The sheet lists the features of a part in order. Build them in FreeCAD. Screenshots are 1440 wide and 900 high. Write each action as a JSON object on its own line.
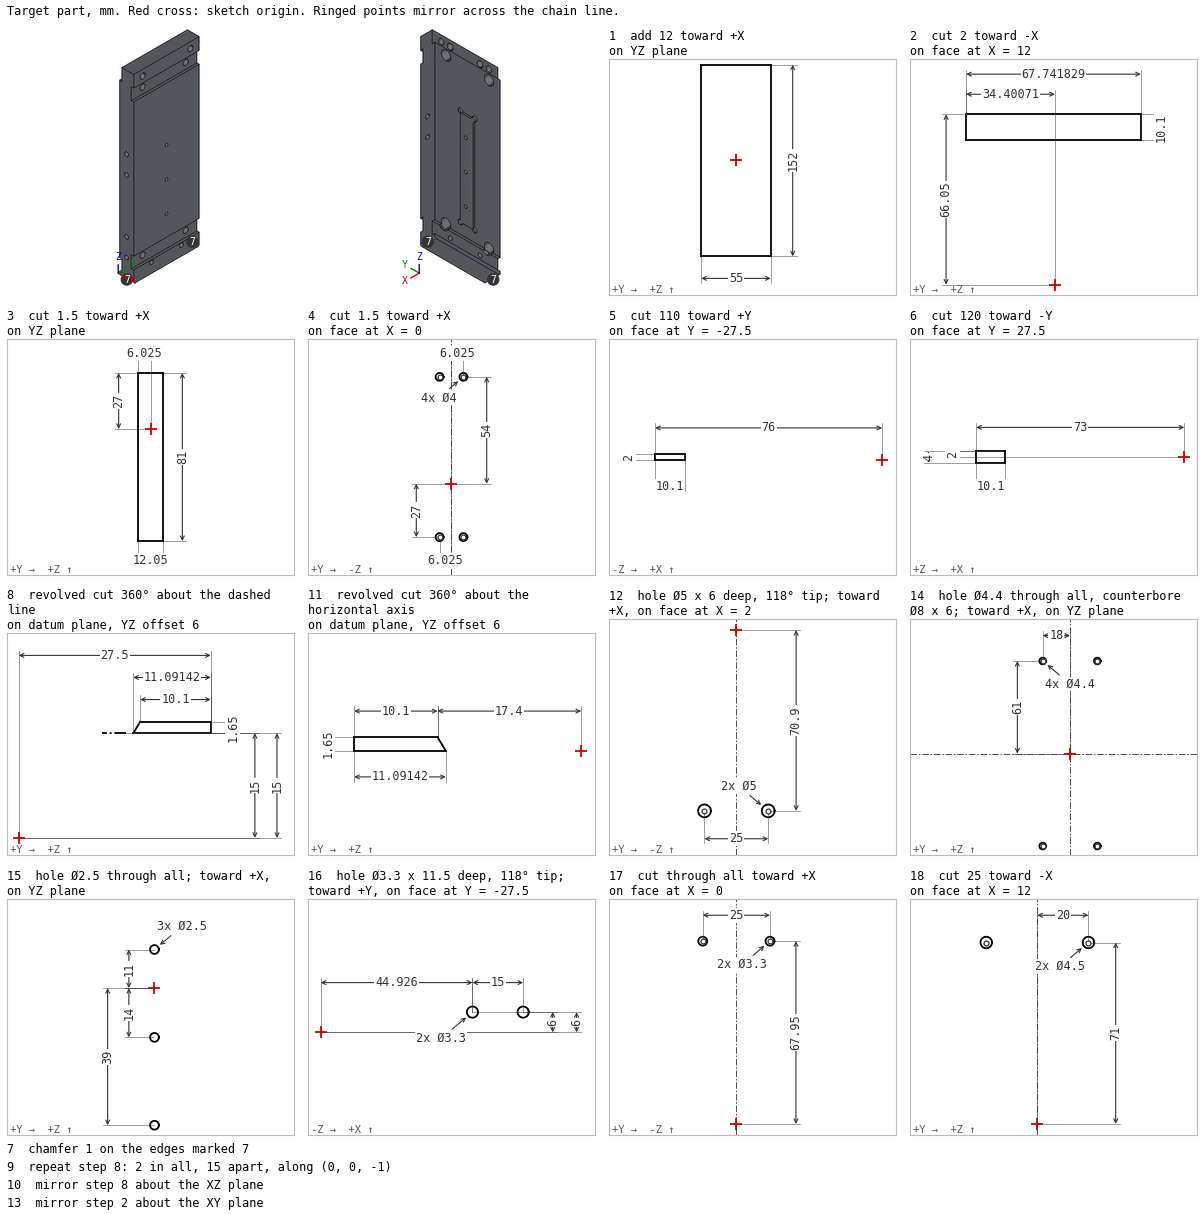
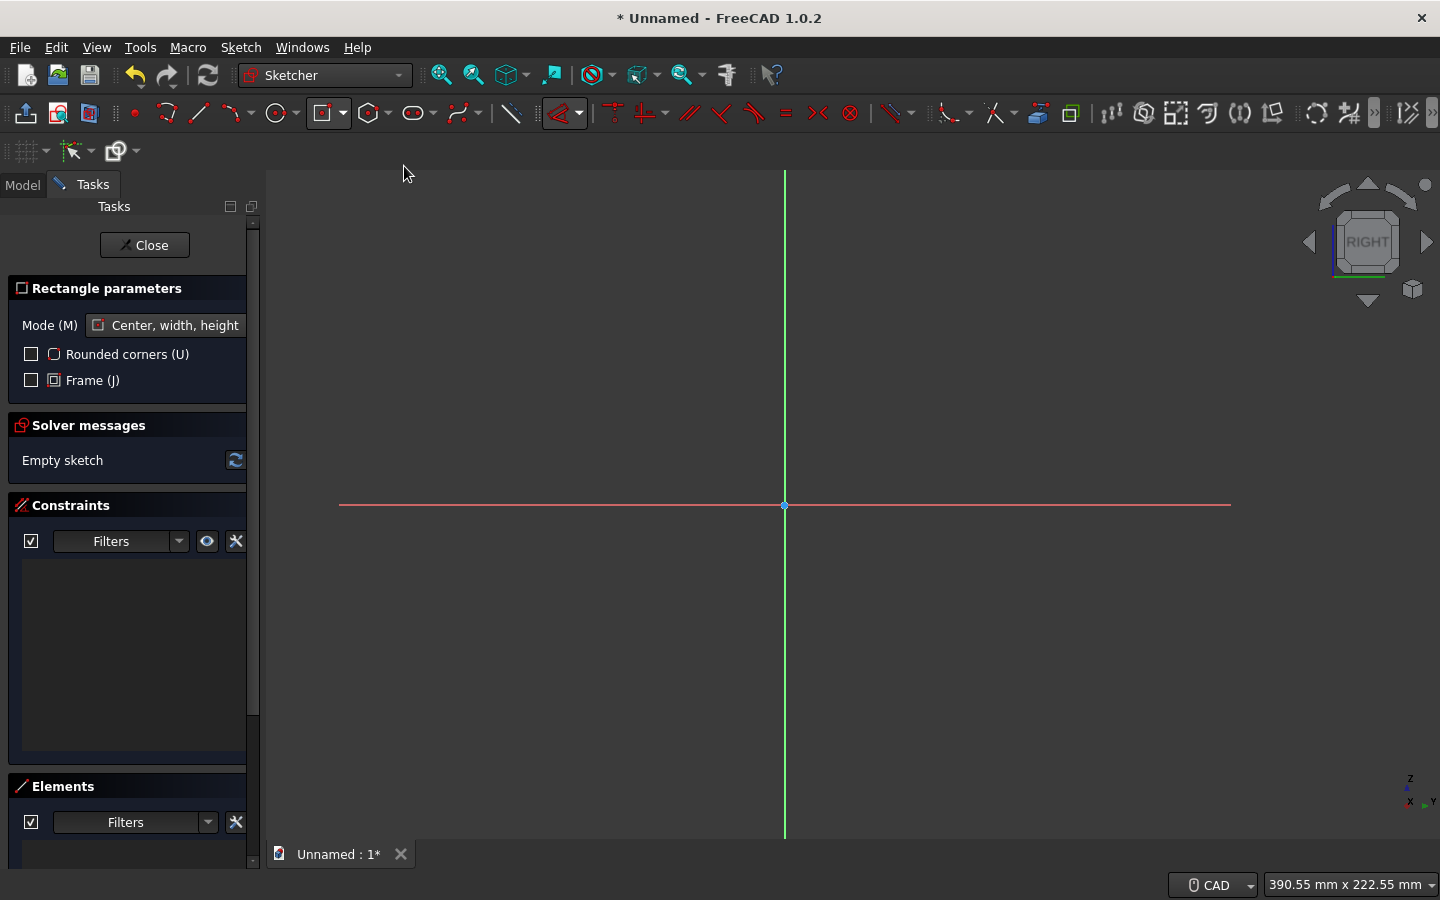
{"action": "left_click", "coordinate": [785, 505]}
{"action": "mouse_move", "coordinate": [868, 277]}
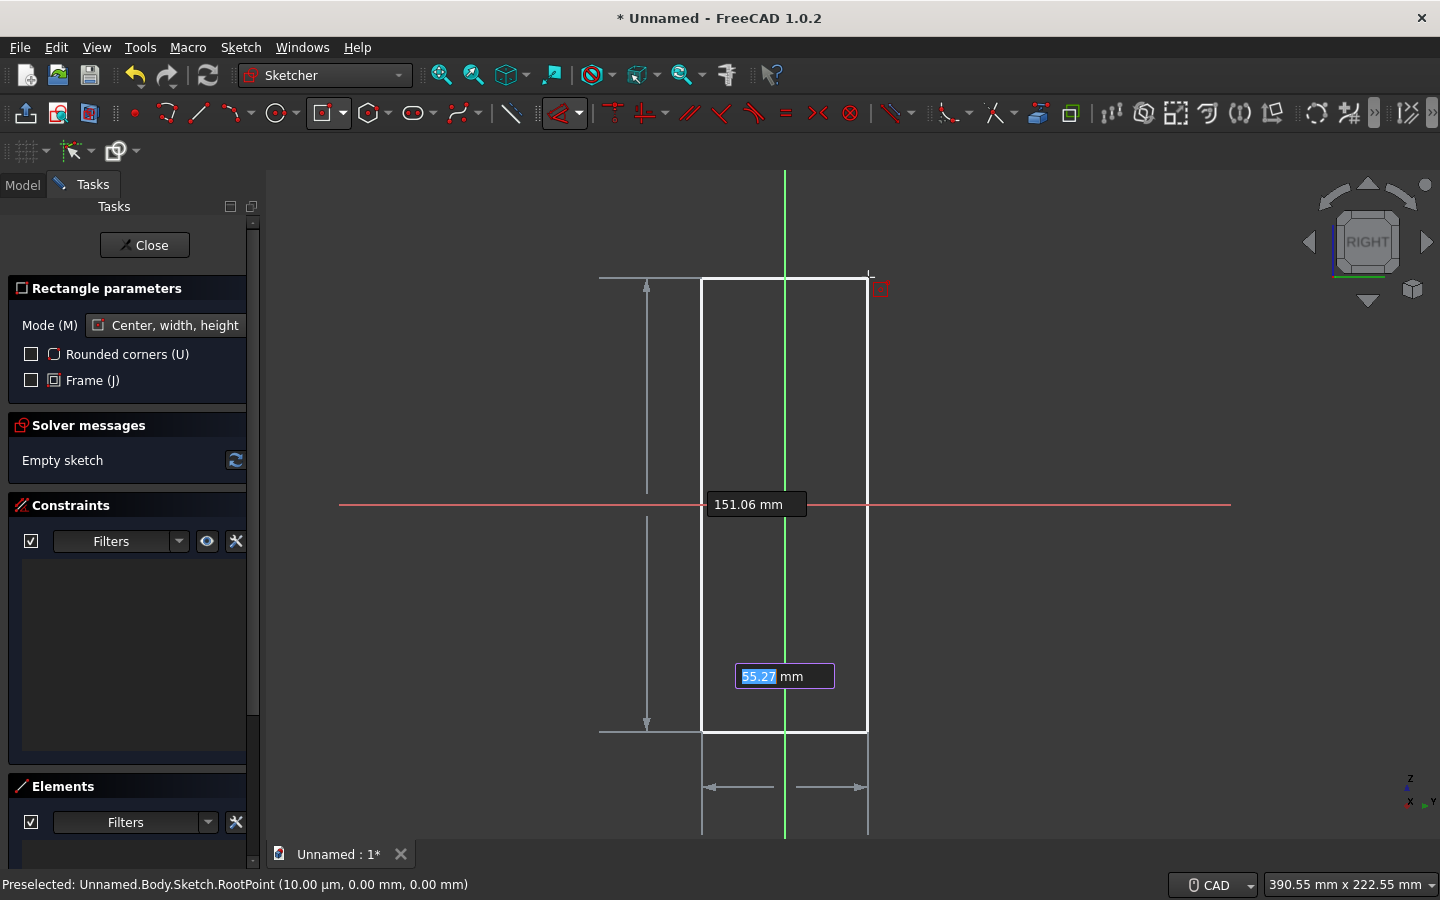
{"action": "type", "text": "55"}
{"action": "key", "text": "Tab"}
{"action": "type", "text": "152"}
{"action": "key", "text": "Return"}
{"action": "key", "text": "Escape"}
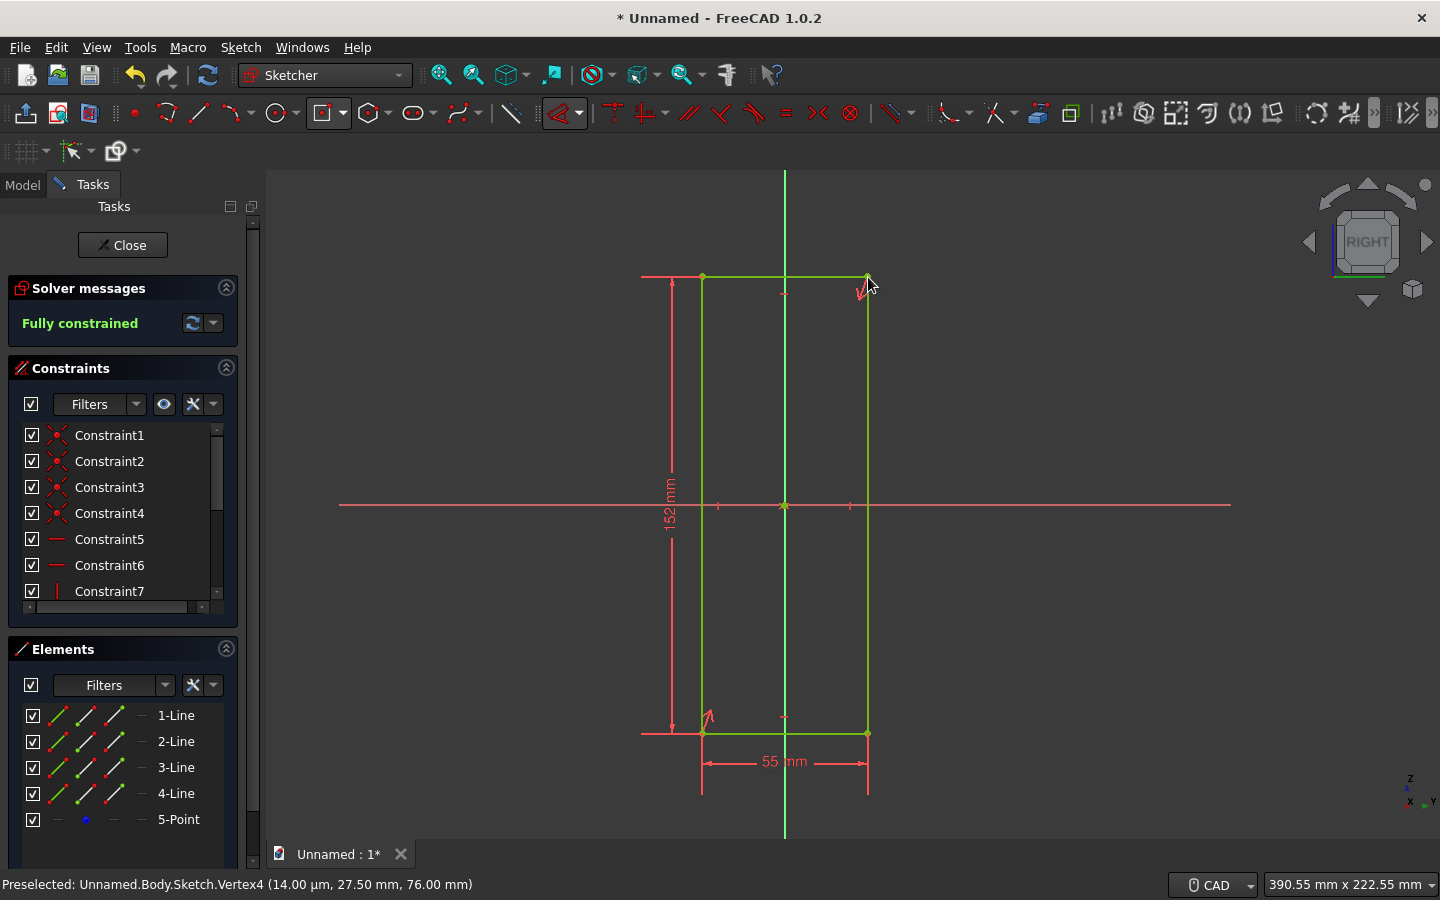
{"action": "left_click", "coordinate": [123, 245]}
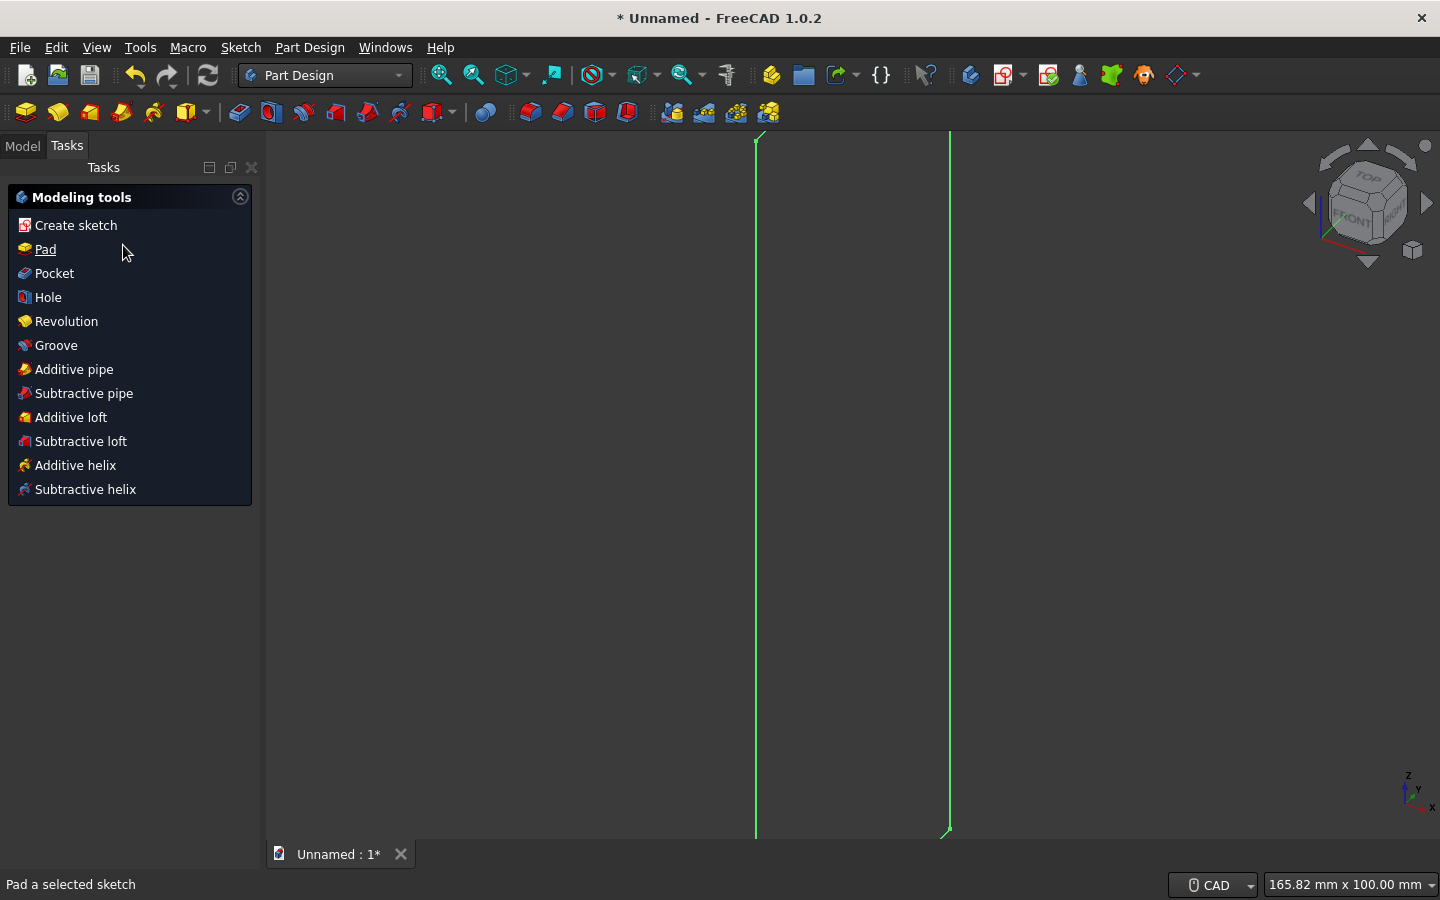
{"action": "left_click", "coordinate": [26, 112]}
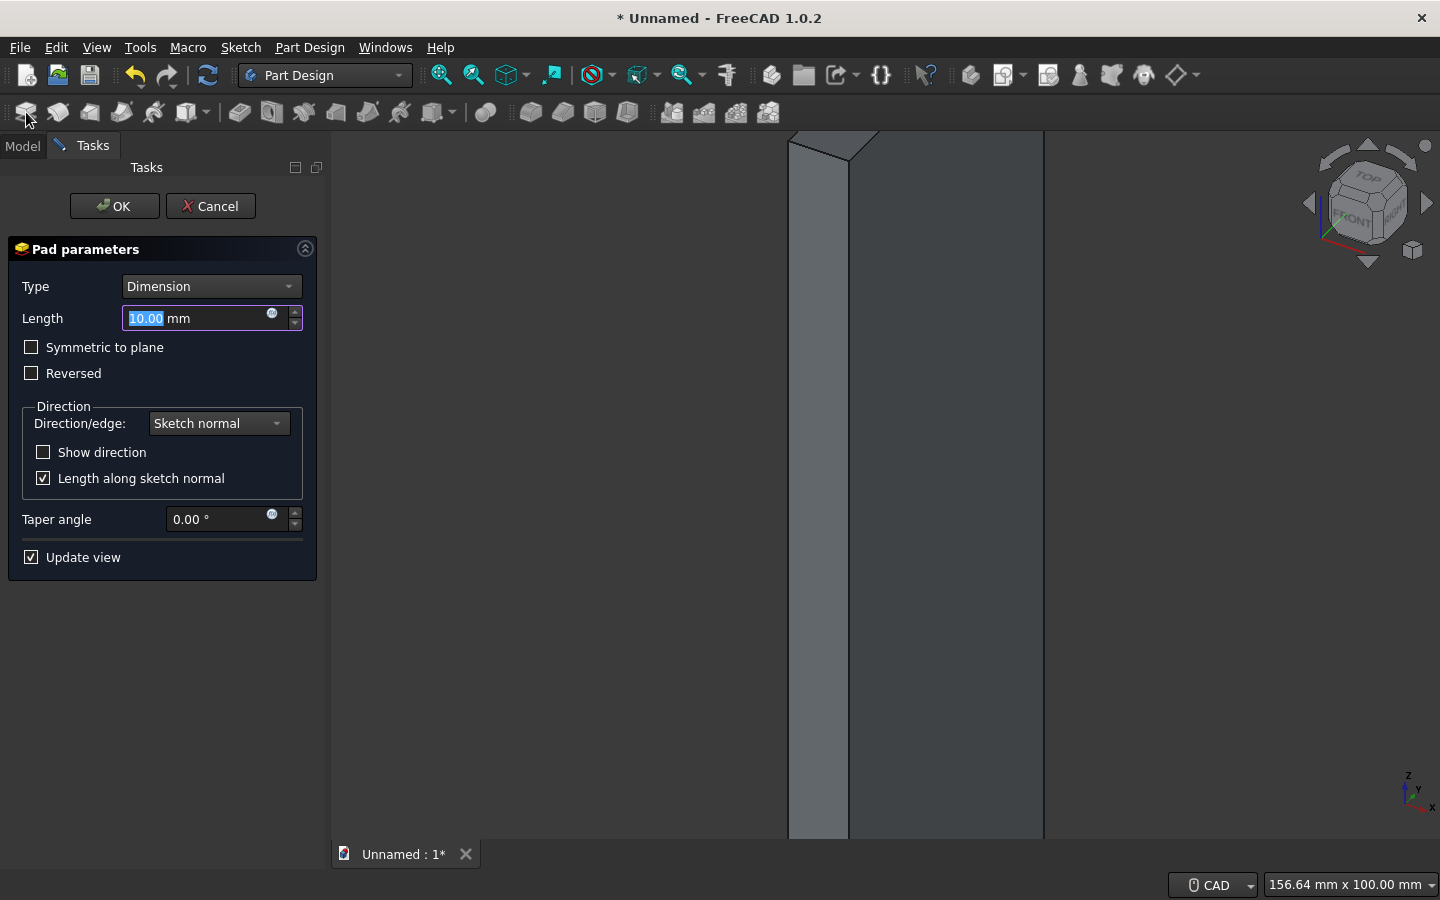
{"action": "type", "text": "12"}
{"action": "key", "text": "Tab"}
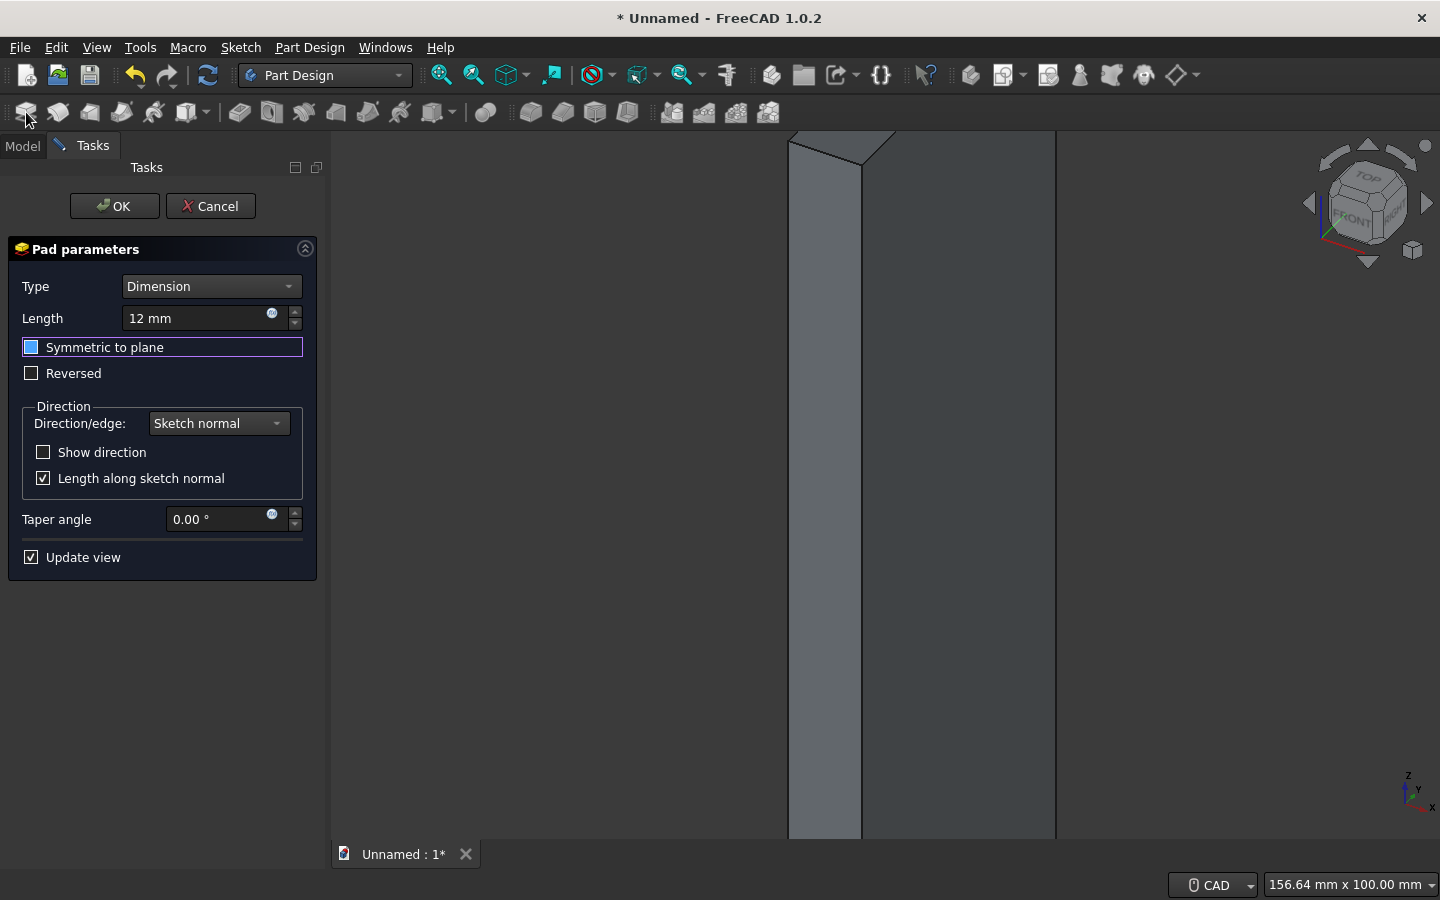
{"action": "left_click", "coordinate": [115, 206]}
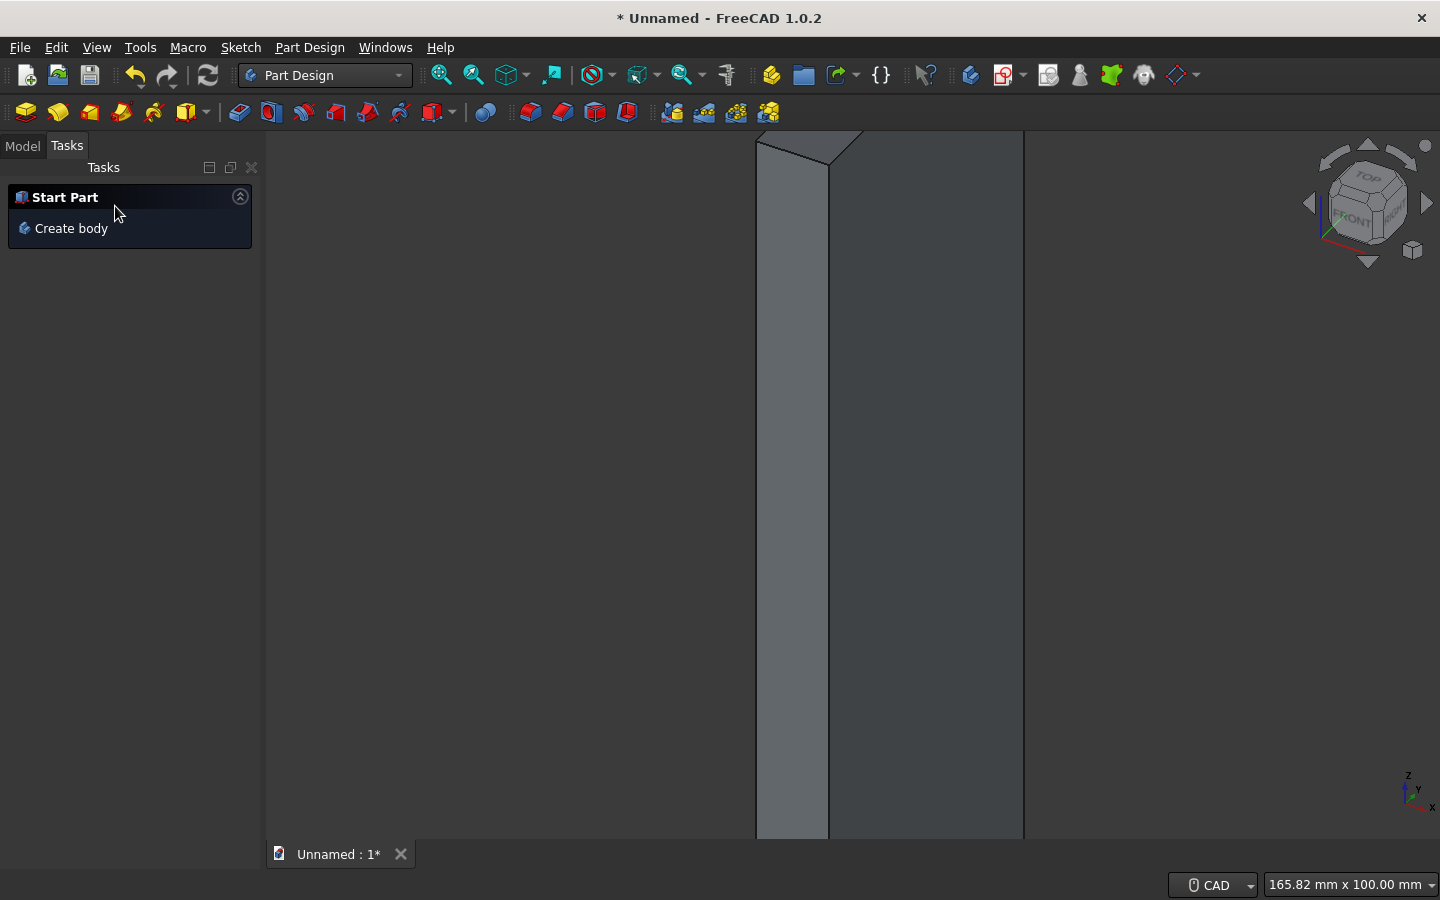
{"action": "left_click", "coordinate": [442, 76]}